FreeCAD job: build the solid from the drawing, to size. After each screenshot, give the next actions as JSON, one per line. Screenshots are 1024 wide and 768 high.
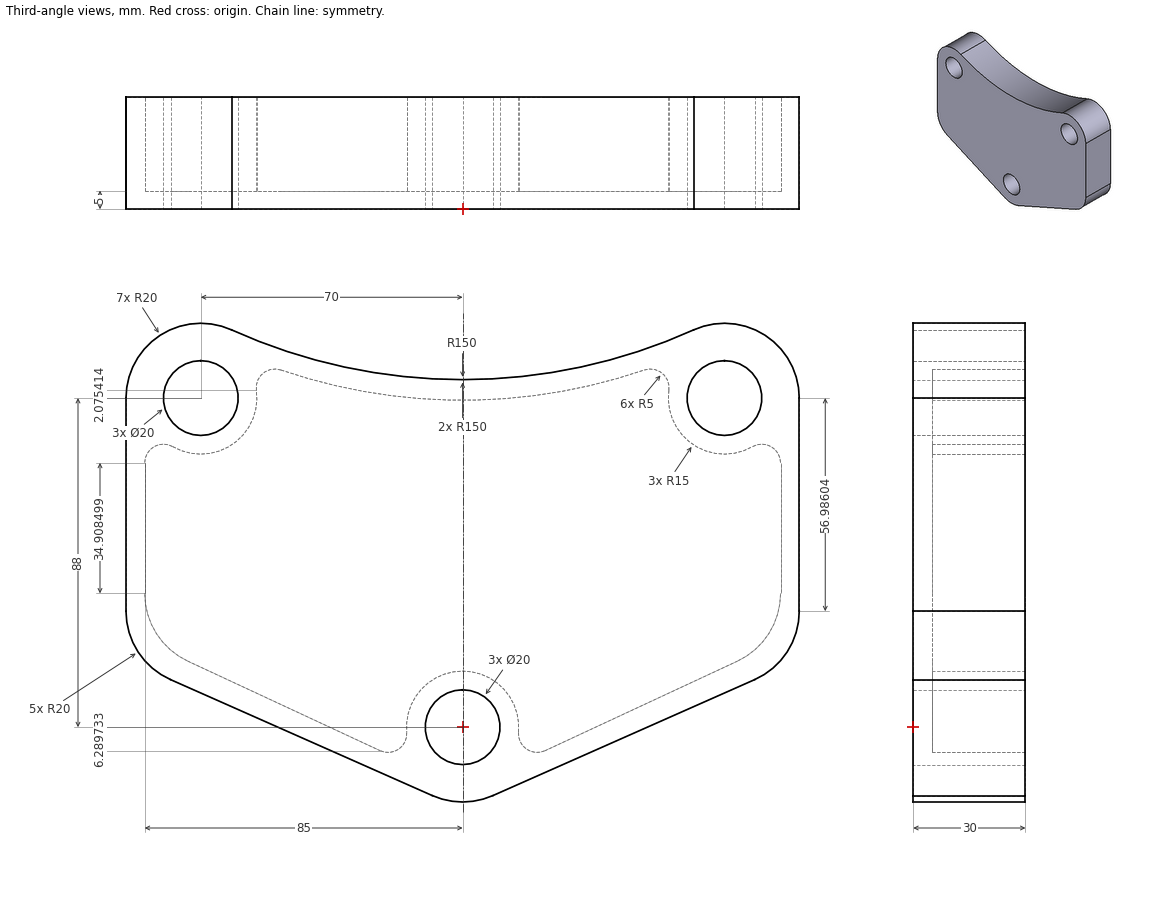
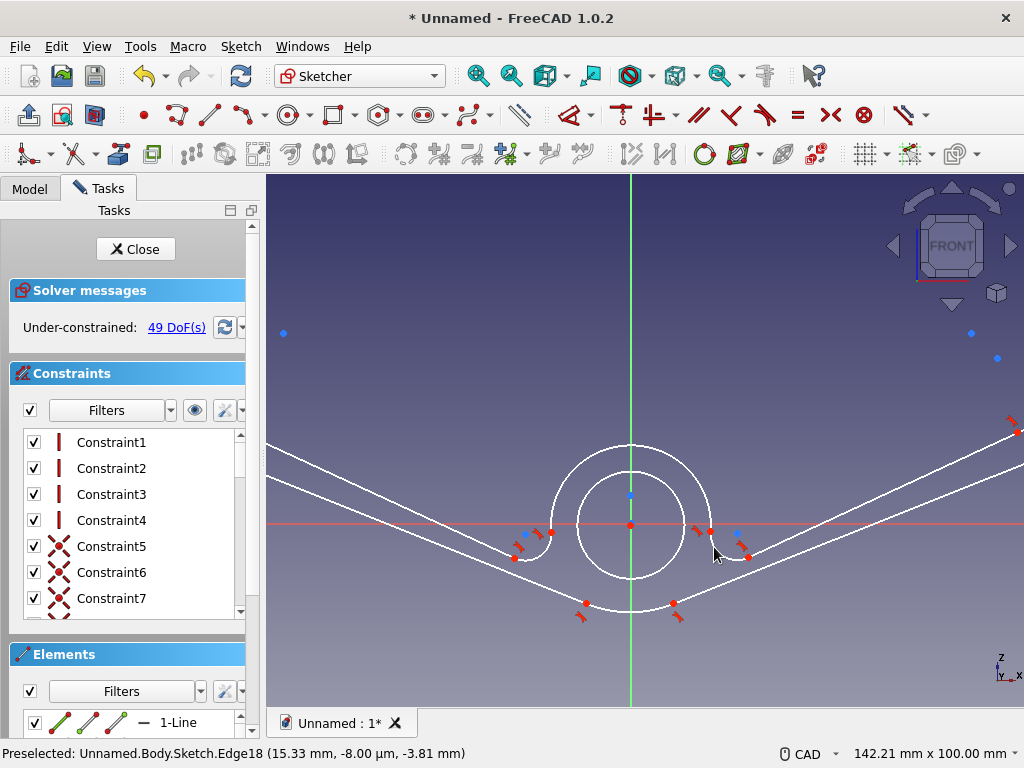
{"action": "scroll", "coordinate": [532, 560], "scroll_direction": "down", "scroll_amount": 4}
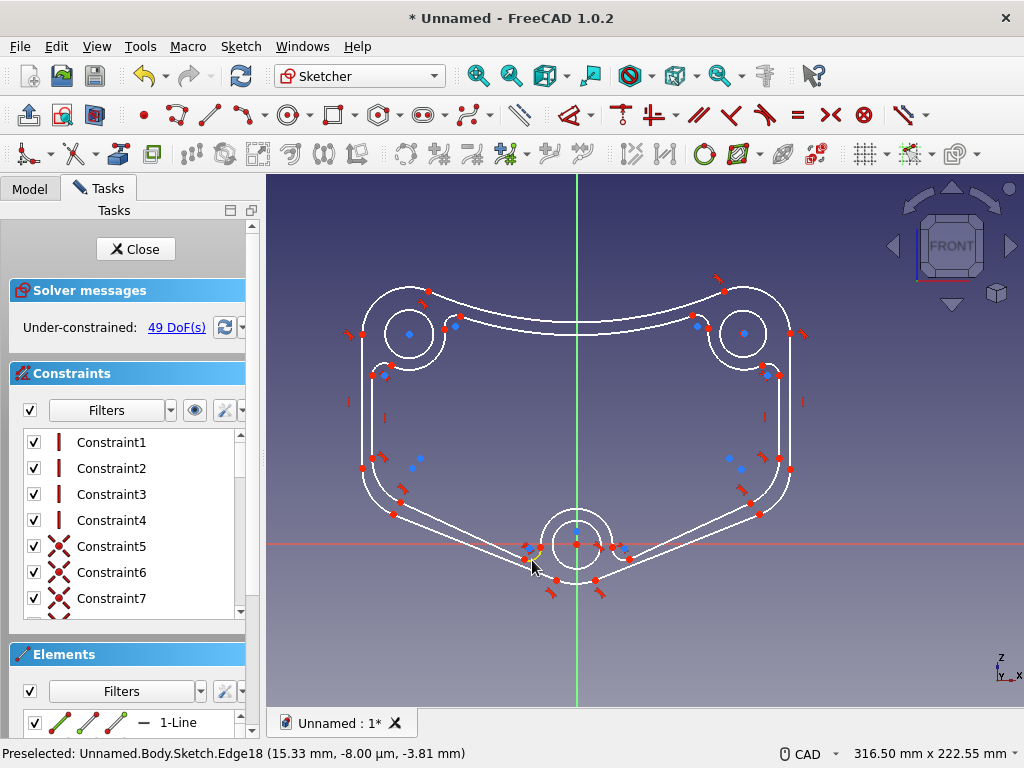
{"action": "scroll", "coordinate": [777, 369], "scroll_direction": "up", "scroll_amount": 4}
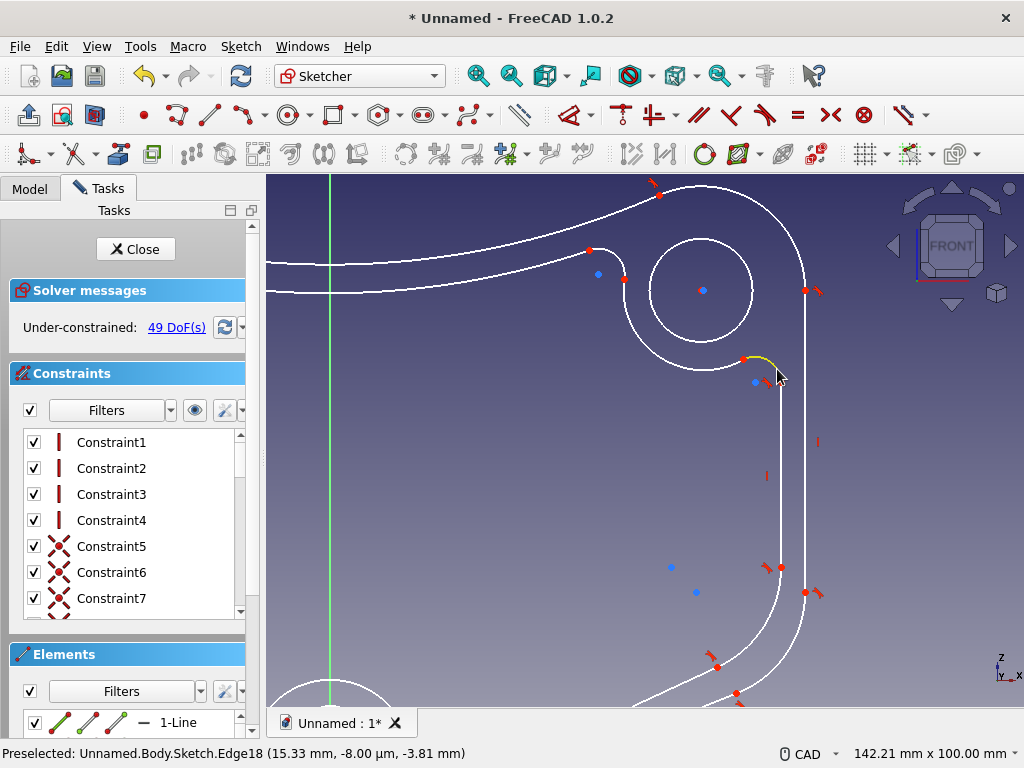
{"action": "left_click", "coordinate": [776, 368]}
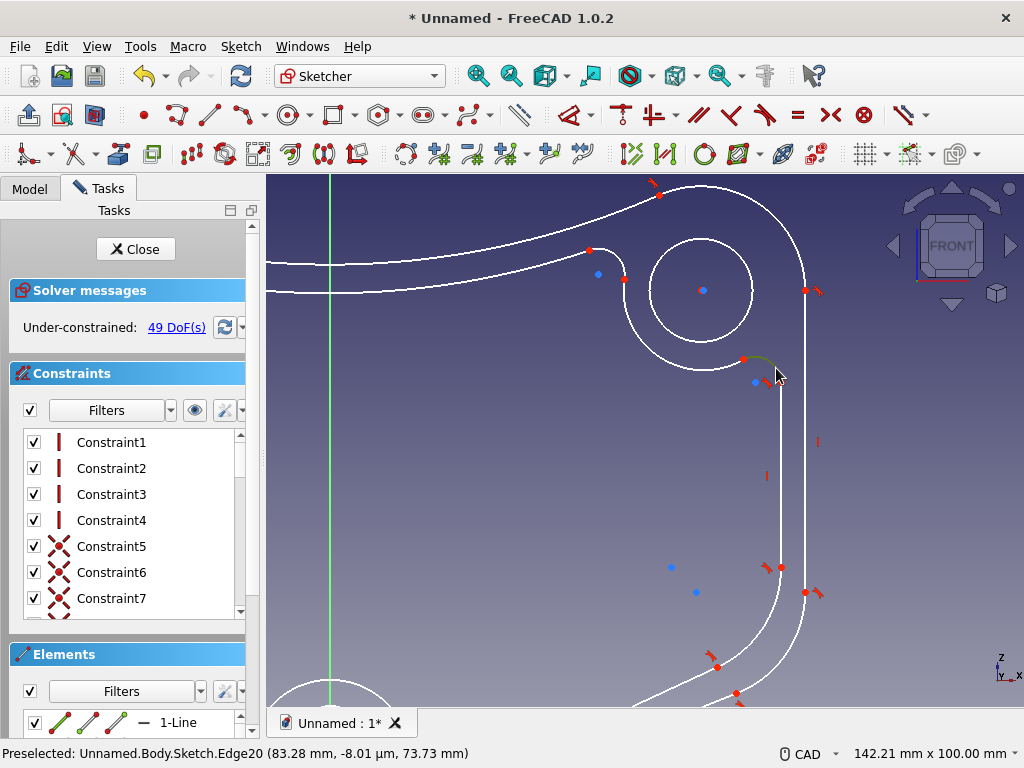
{"action": "left_click", "coordinate": [635, 331]}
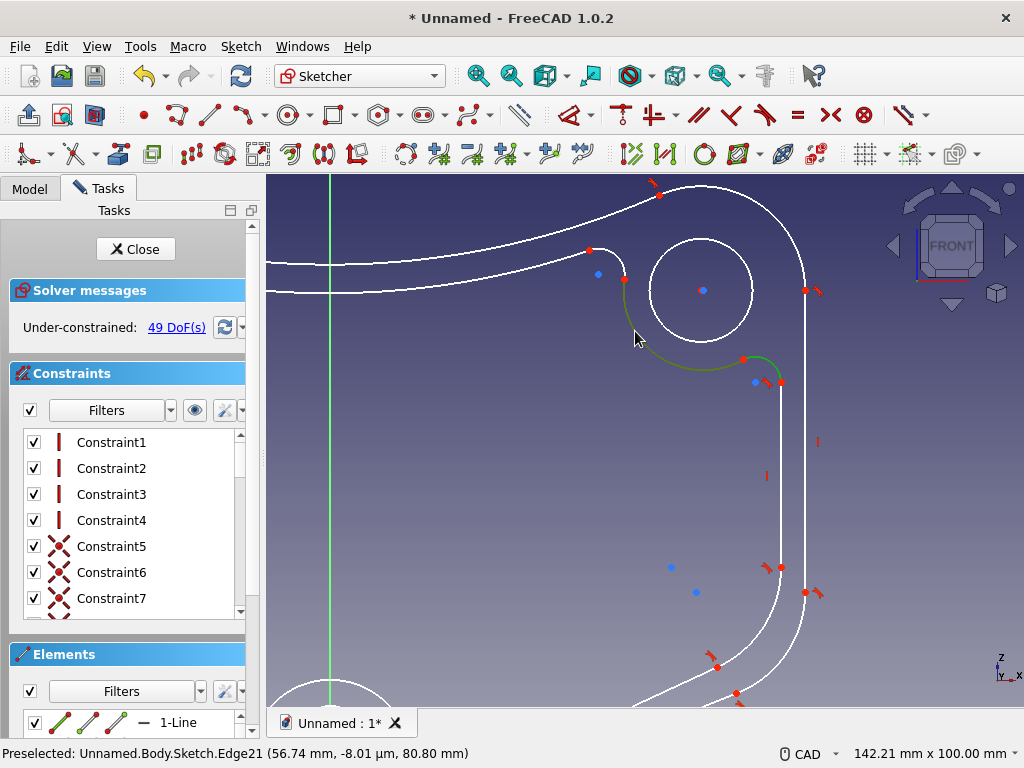
{"action": "key", "text": "t"}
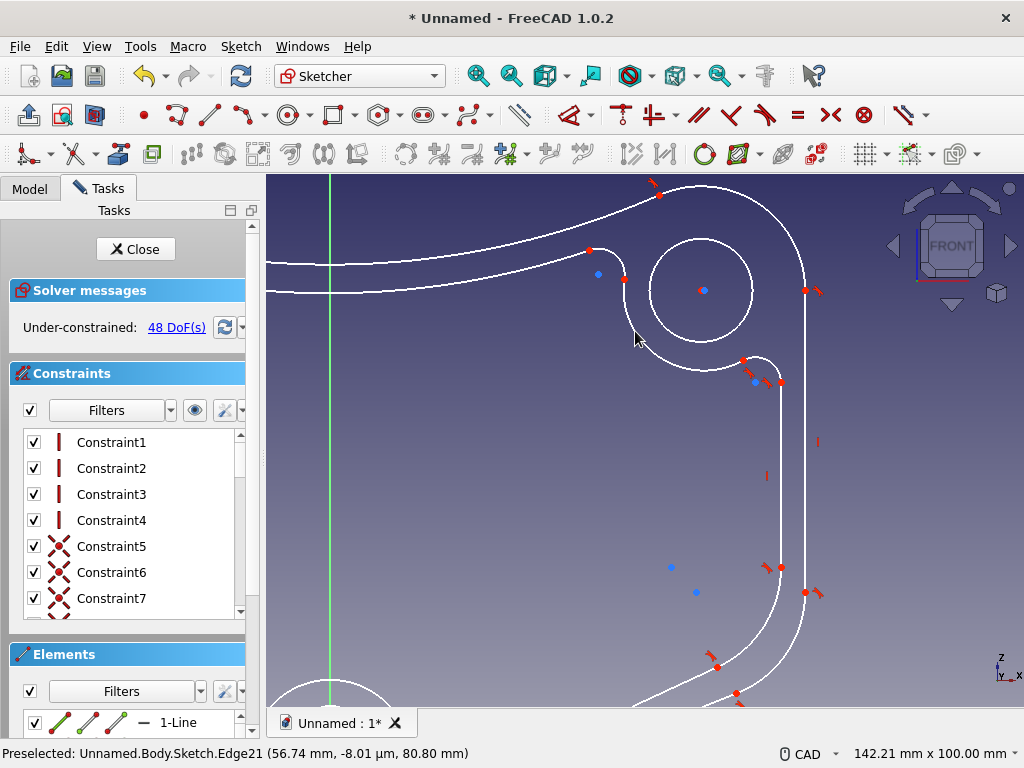
{"action": "left_click", "coordinate": [635, 331]}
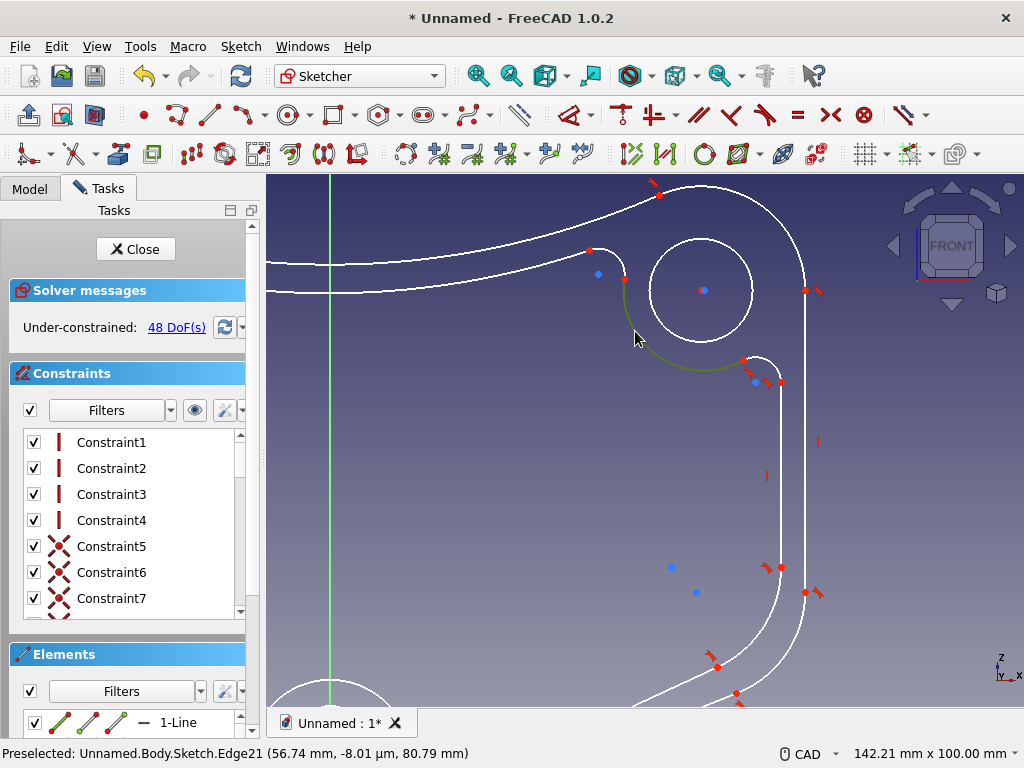
{"action": "left_click", "coordinate": [622, 263]}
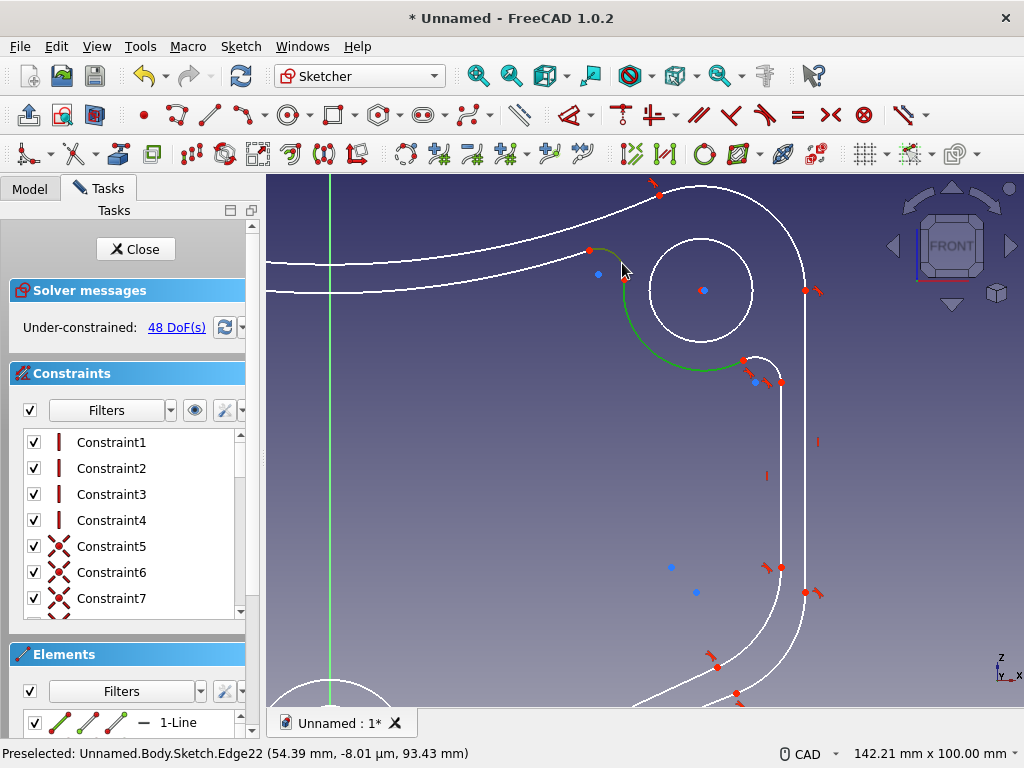
{"action": "left_click", "coordinate": [765, 116]}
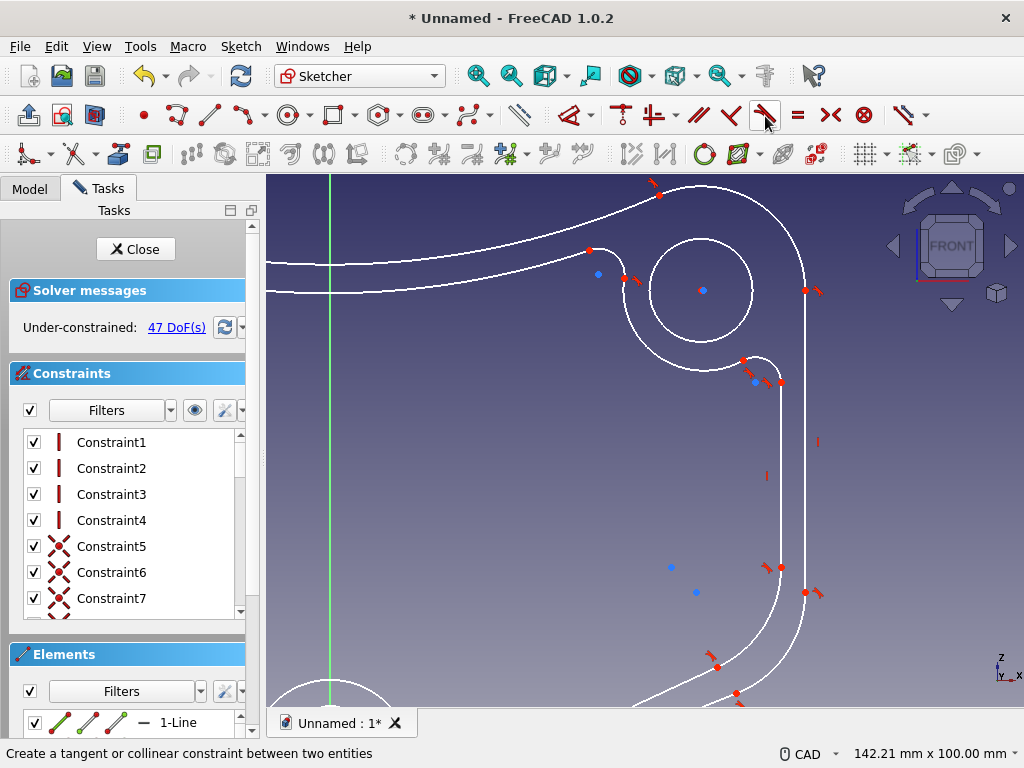
{"action": "left_click", "coordinate": [622, 263]}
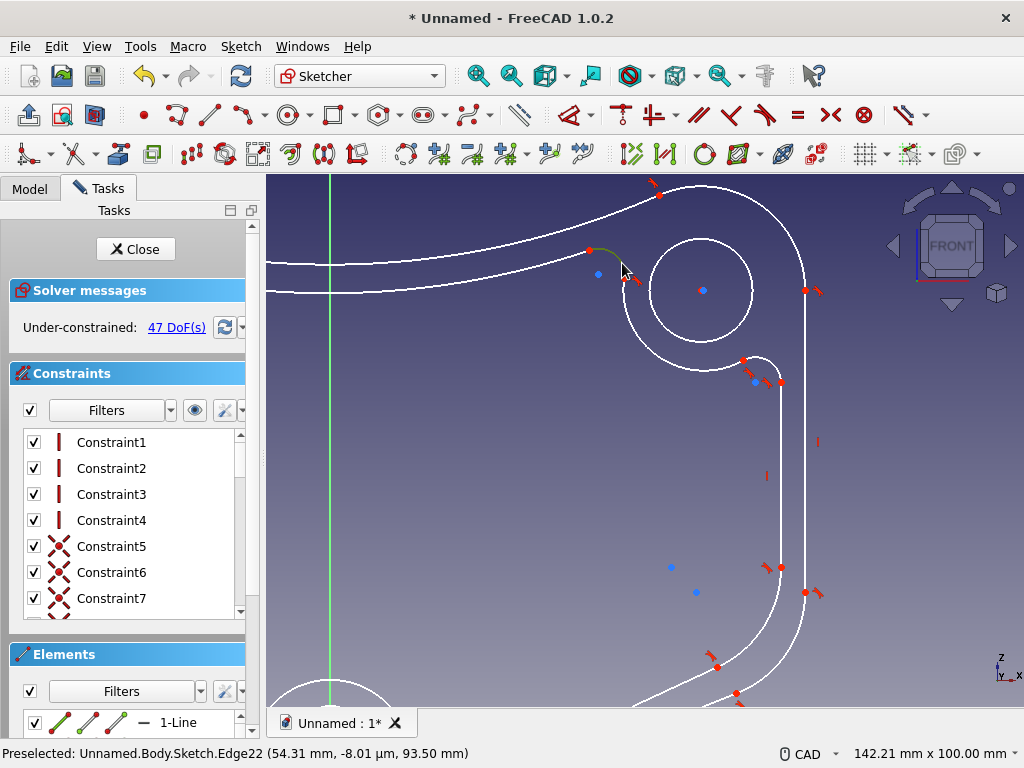
{"action": "left_click", "coordinate": [435, 286]}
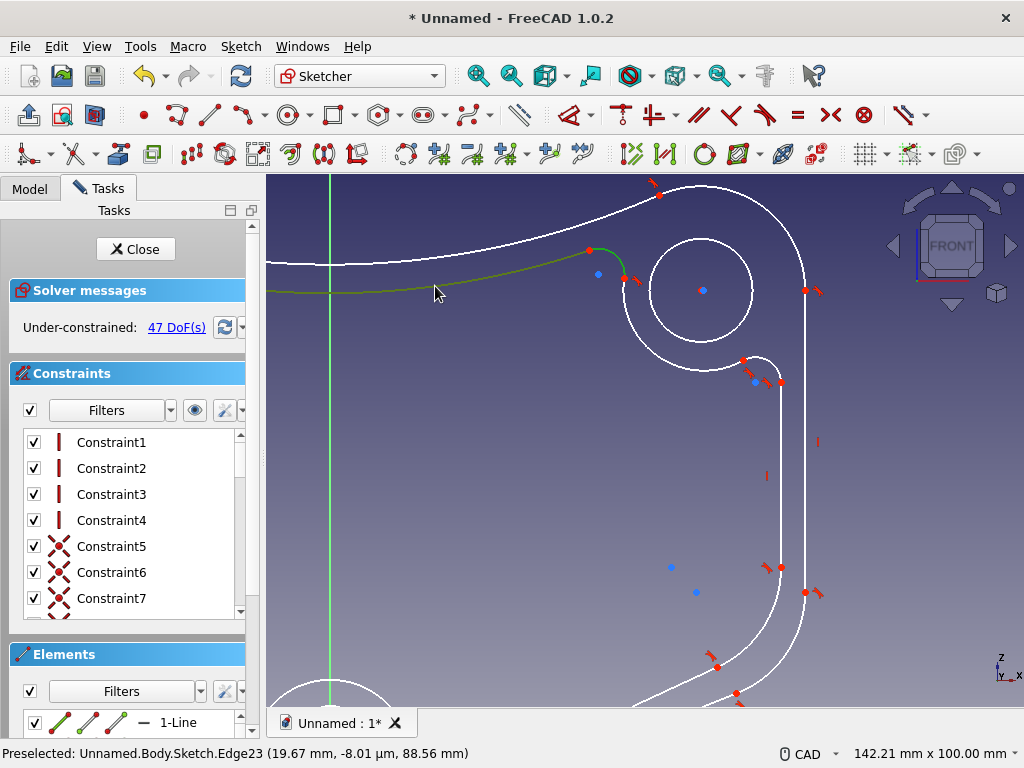
{"action": "left_click", "coordinate": [765, 116]}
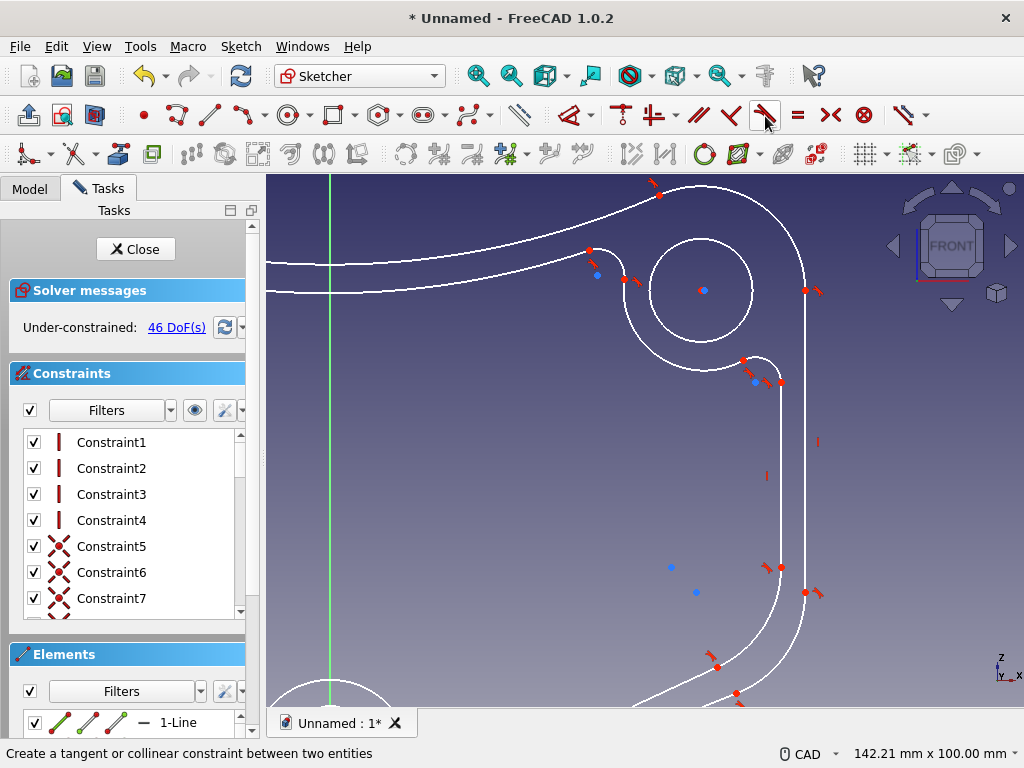
{"action": "left_click", "coordinate": [435, 286]}